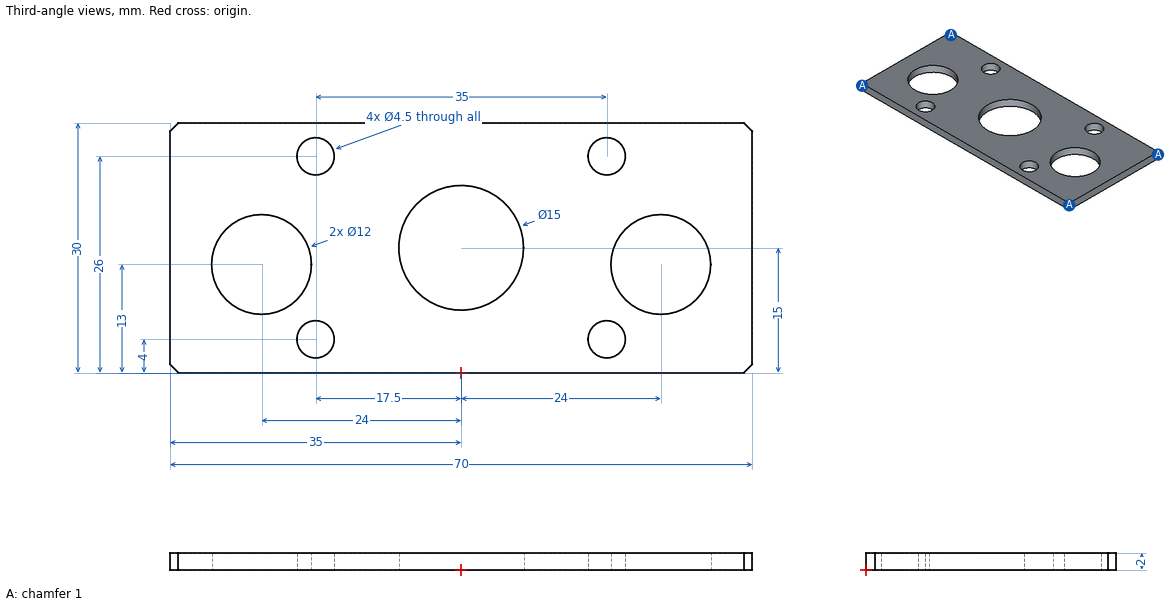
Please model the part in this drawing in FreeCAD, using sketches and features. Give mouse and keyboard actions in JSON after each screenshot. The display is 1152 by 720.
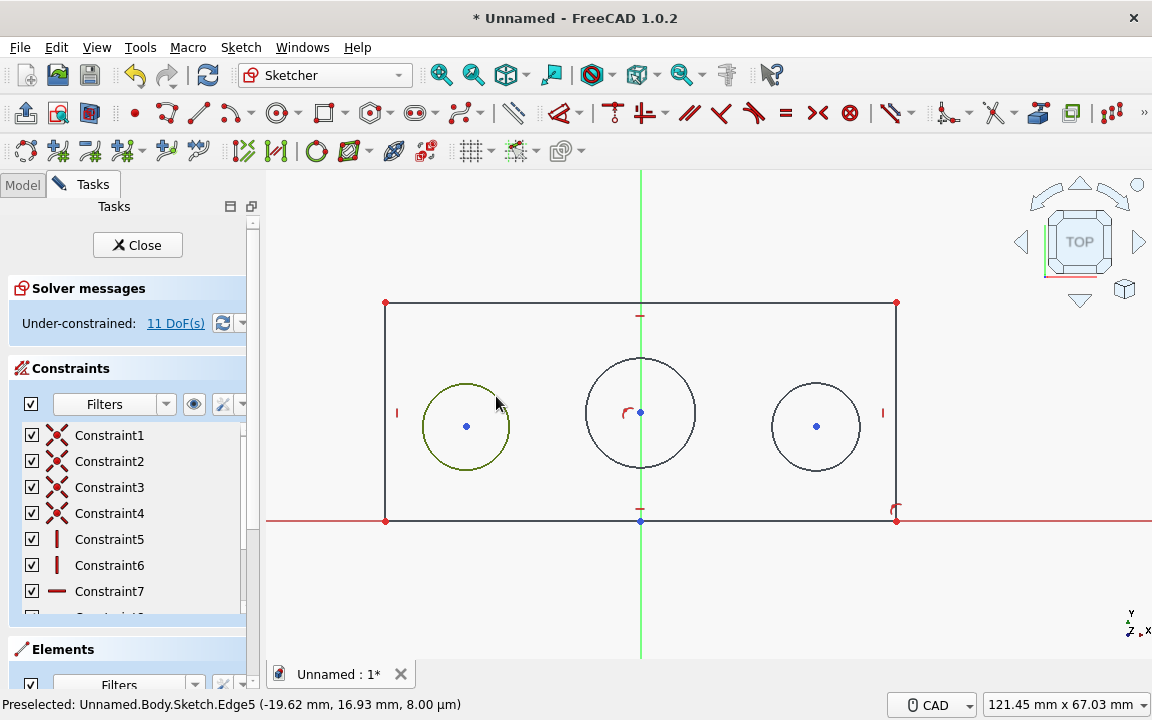
{"action": "left_click", "coordinate": [847, 396]}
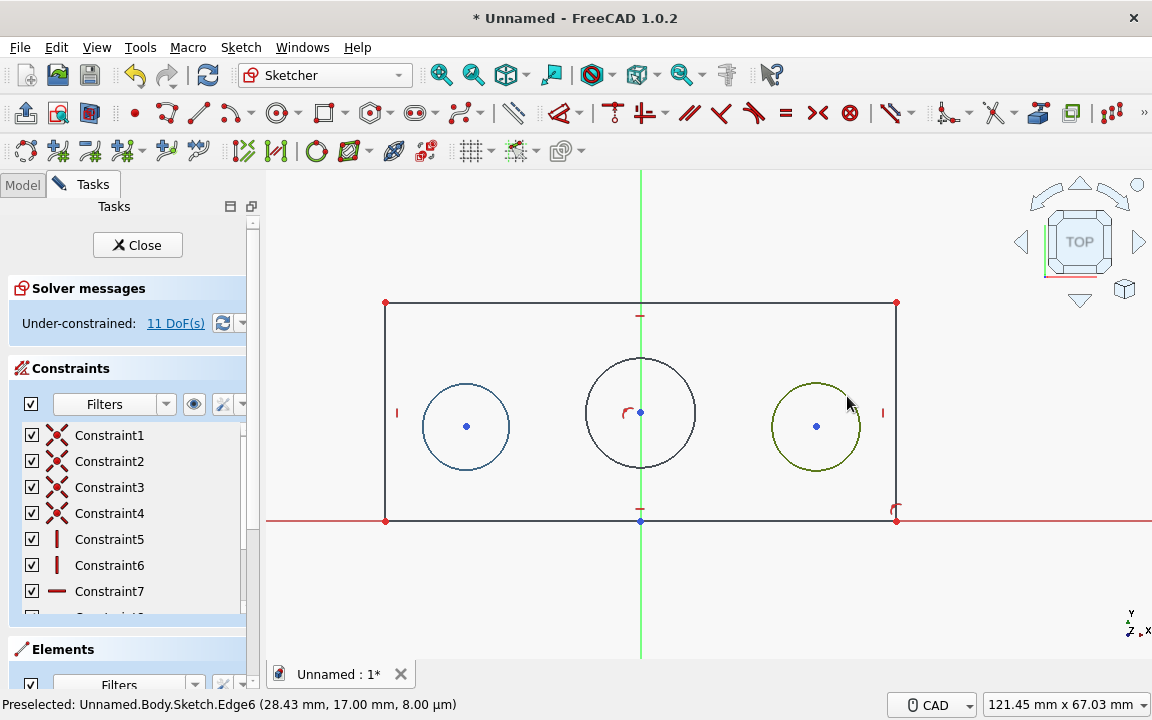
{"action": "left_click", "coordinate": [786, 114]}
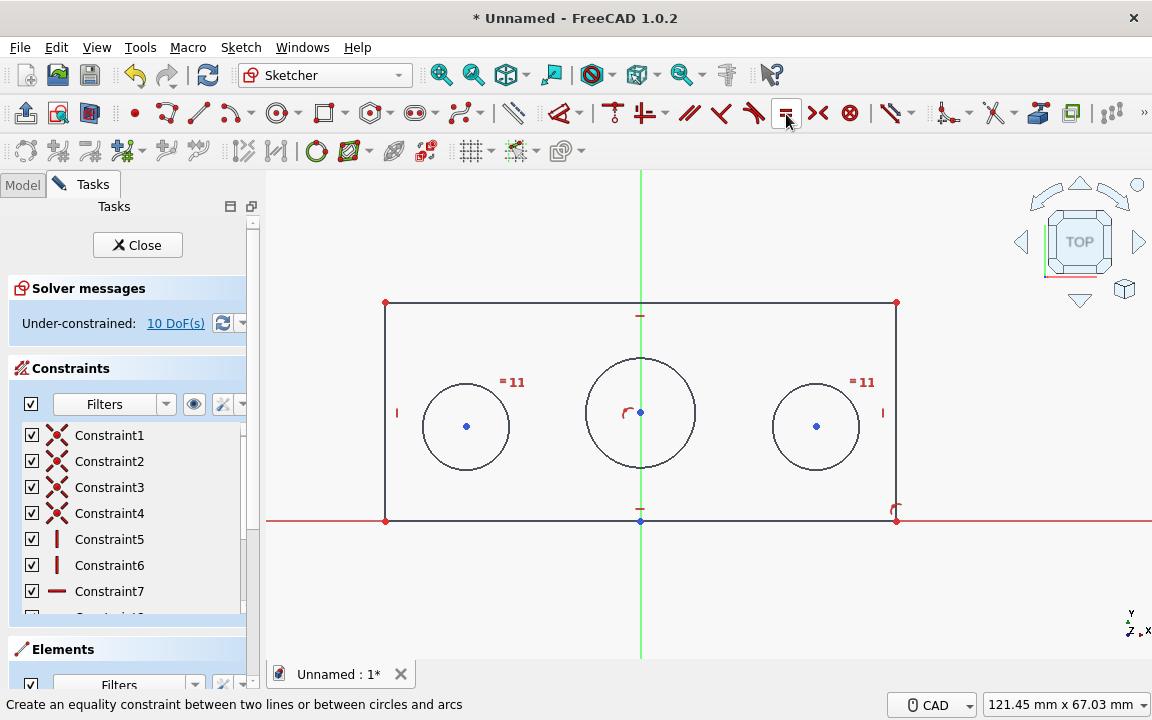
{"action": "left_click", "coordinate": [466, 427]}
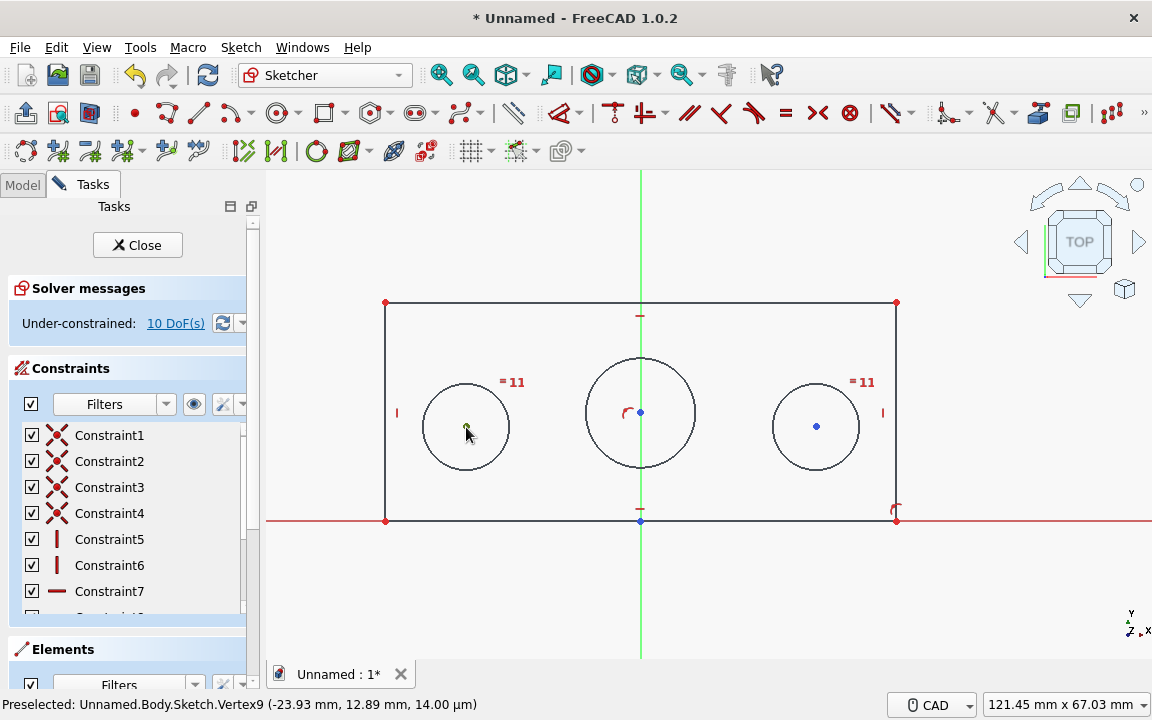
{"action": "left_click", "coordinate": [816, 427]}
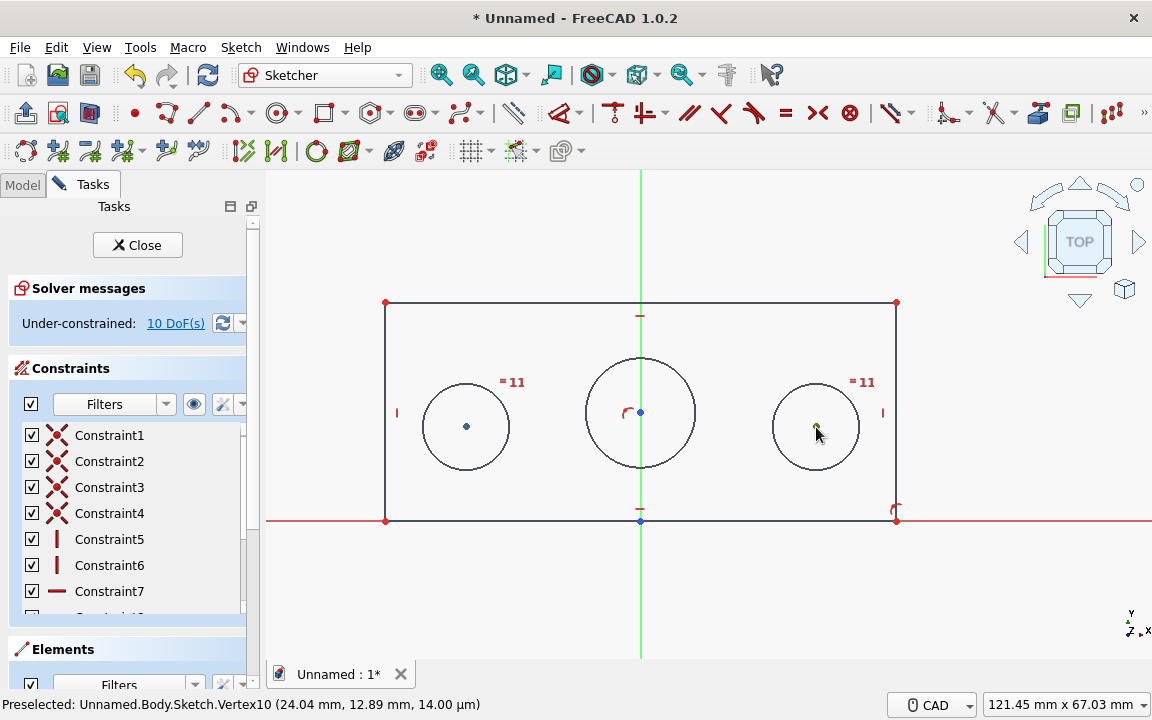
{"action": "key", "text": "h"}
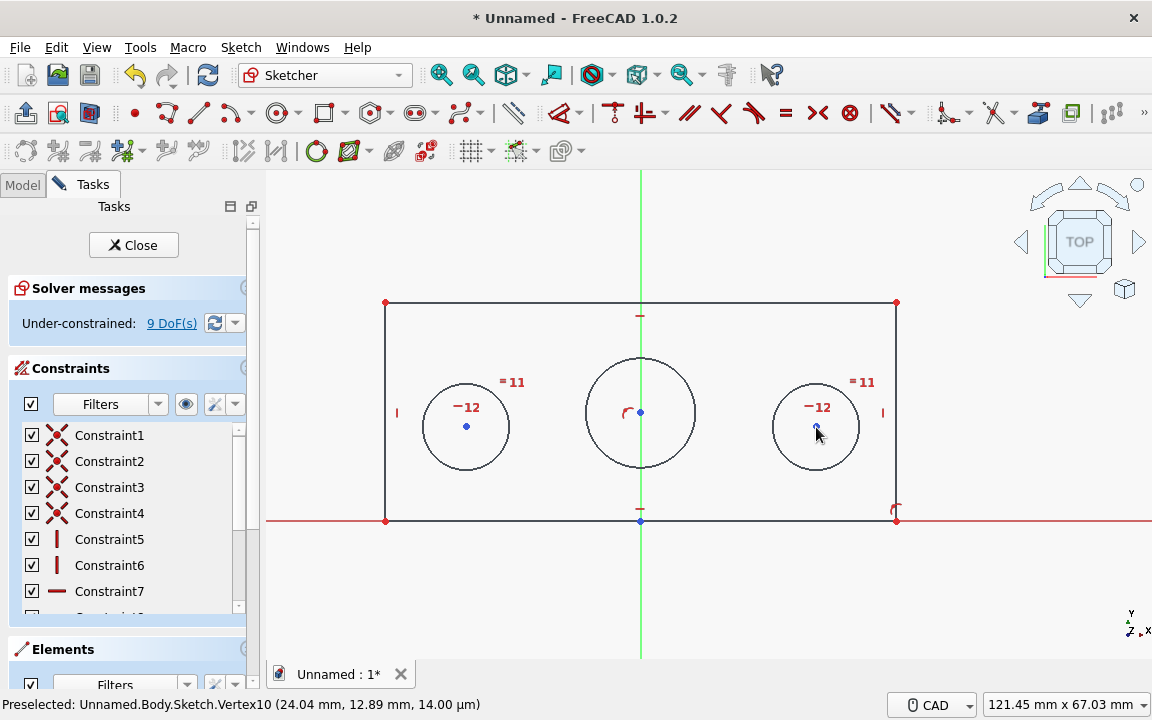
{"action": "left_click", "coordinate": [496, 396]}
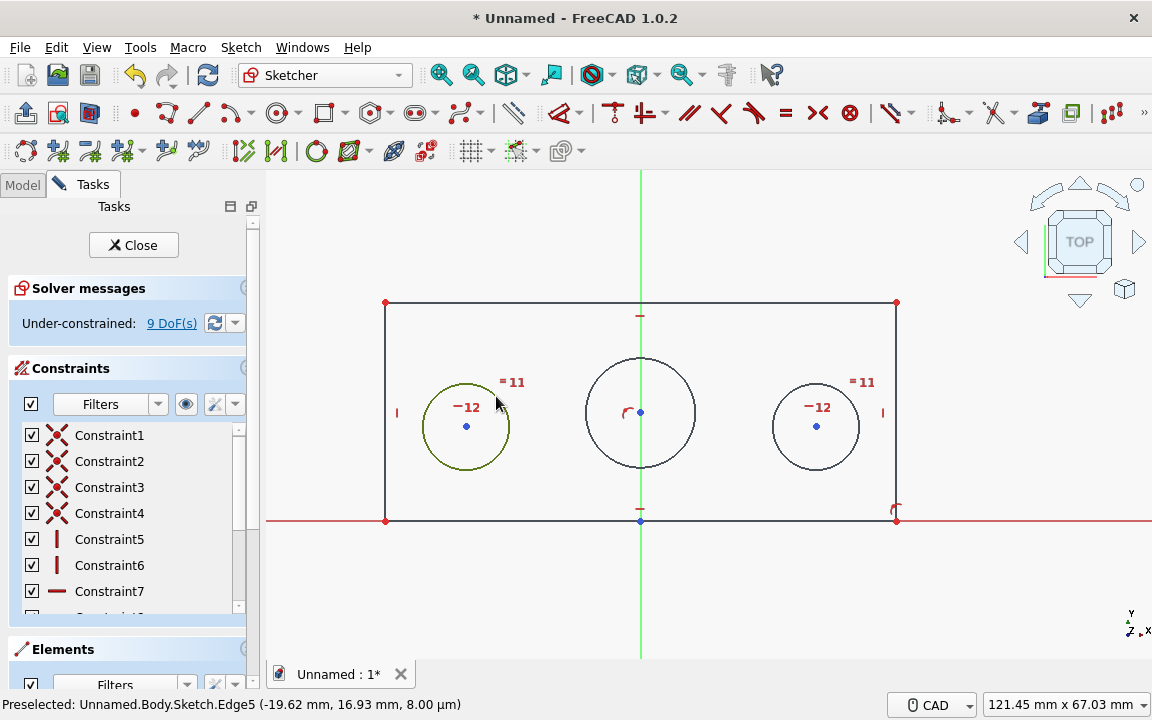
{"action": "left_click", "coordinate": [582, 114]}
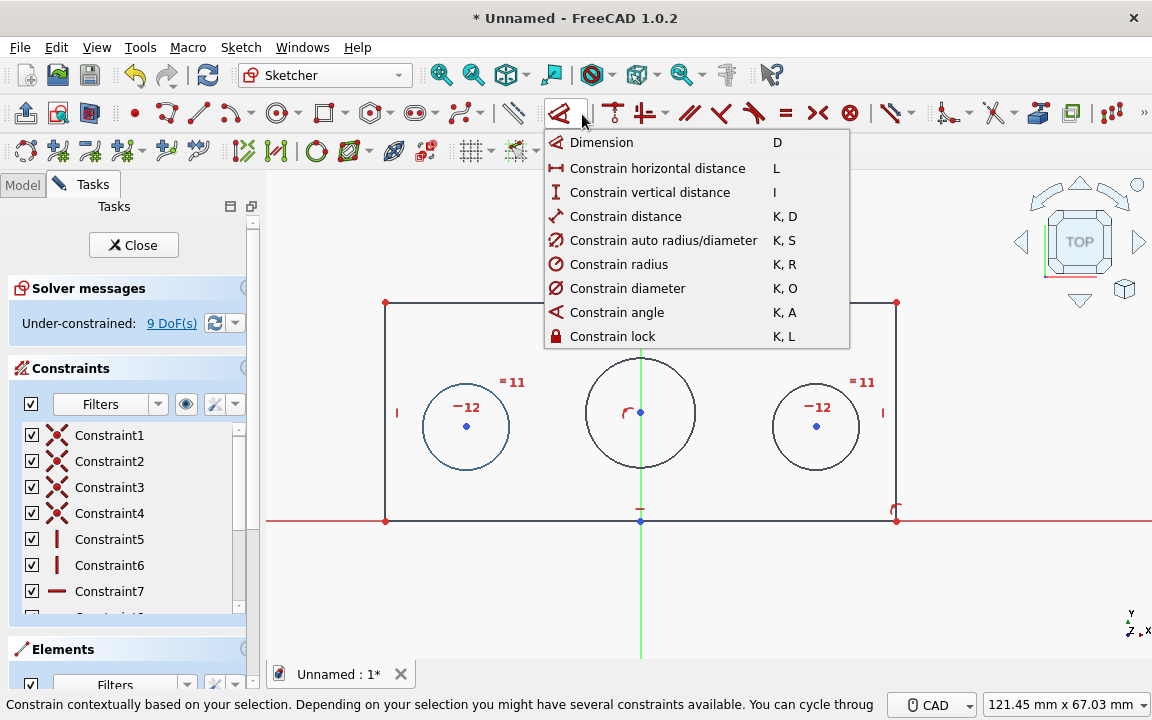
{"action": "left_click", "coordinate": [697, 288]}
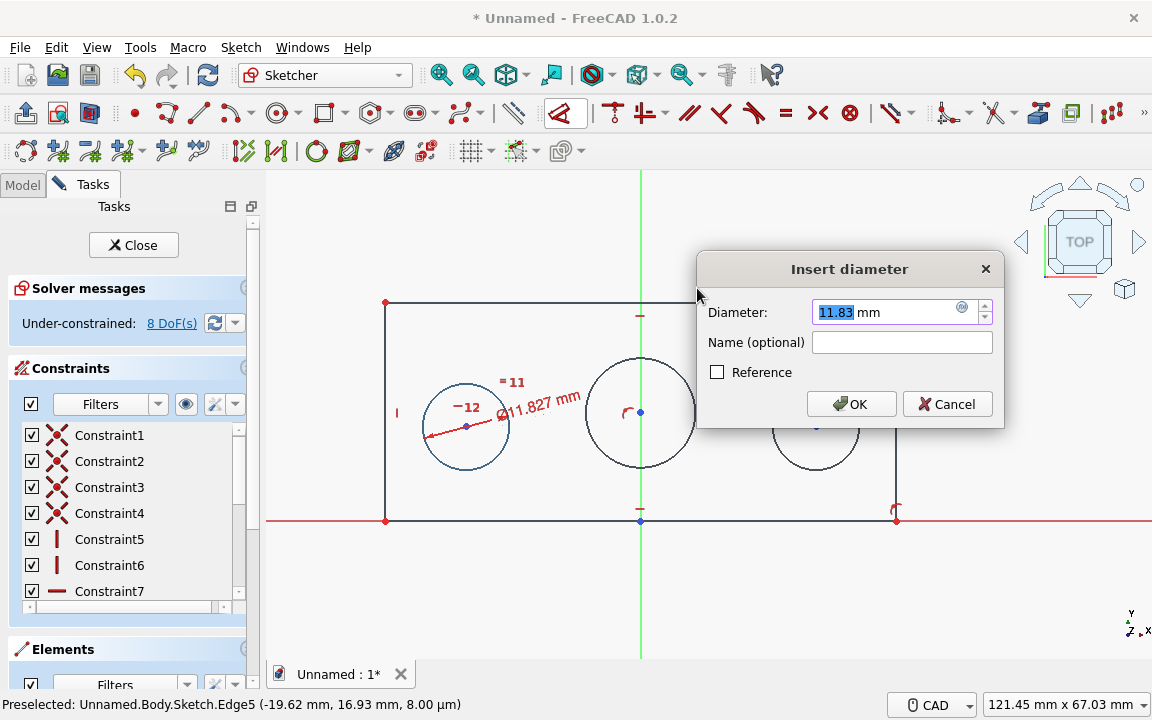
{"action": "type", "text": "12"}
{"action": "key", "text": "Return"}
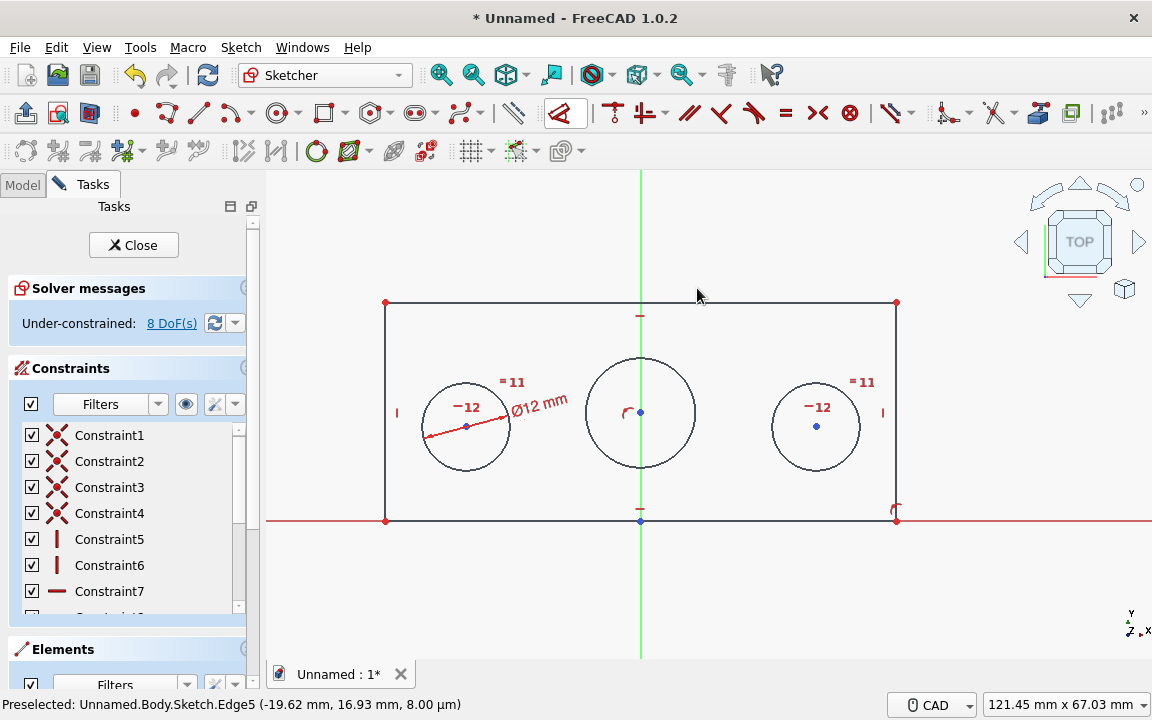
{"action": "left_click", "coordinate": [679, 374]}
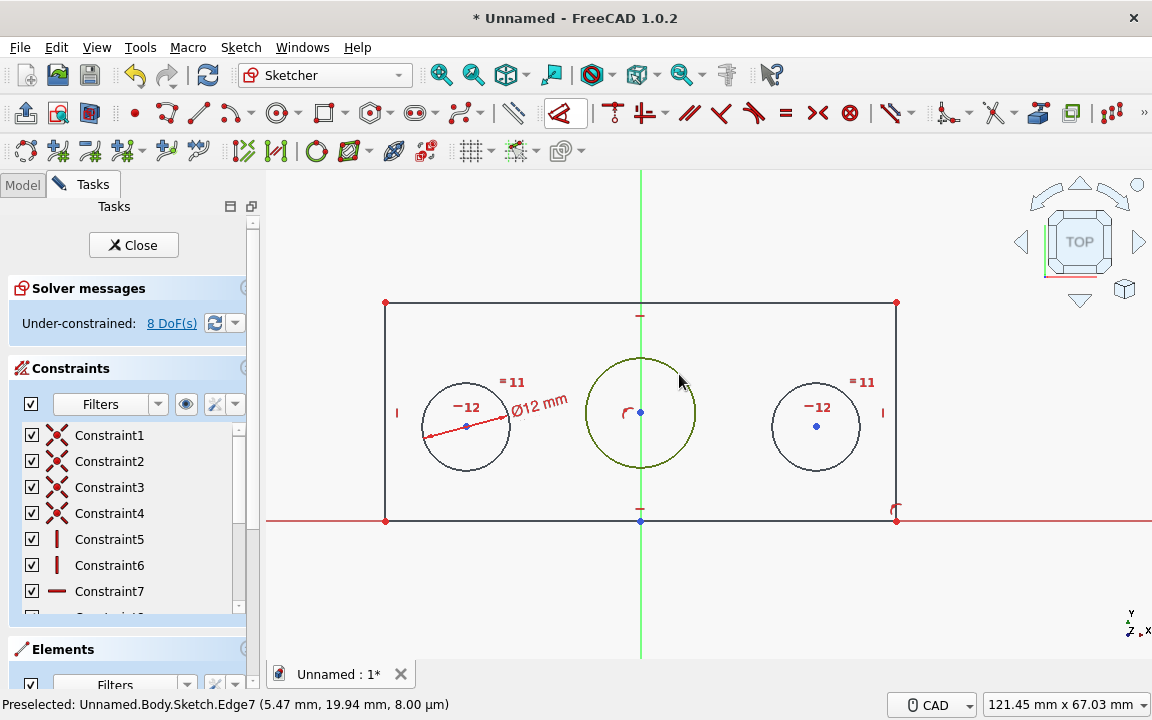
{"action": "left_click", "coordinate": [582, 114]}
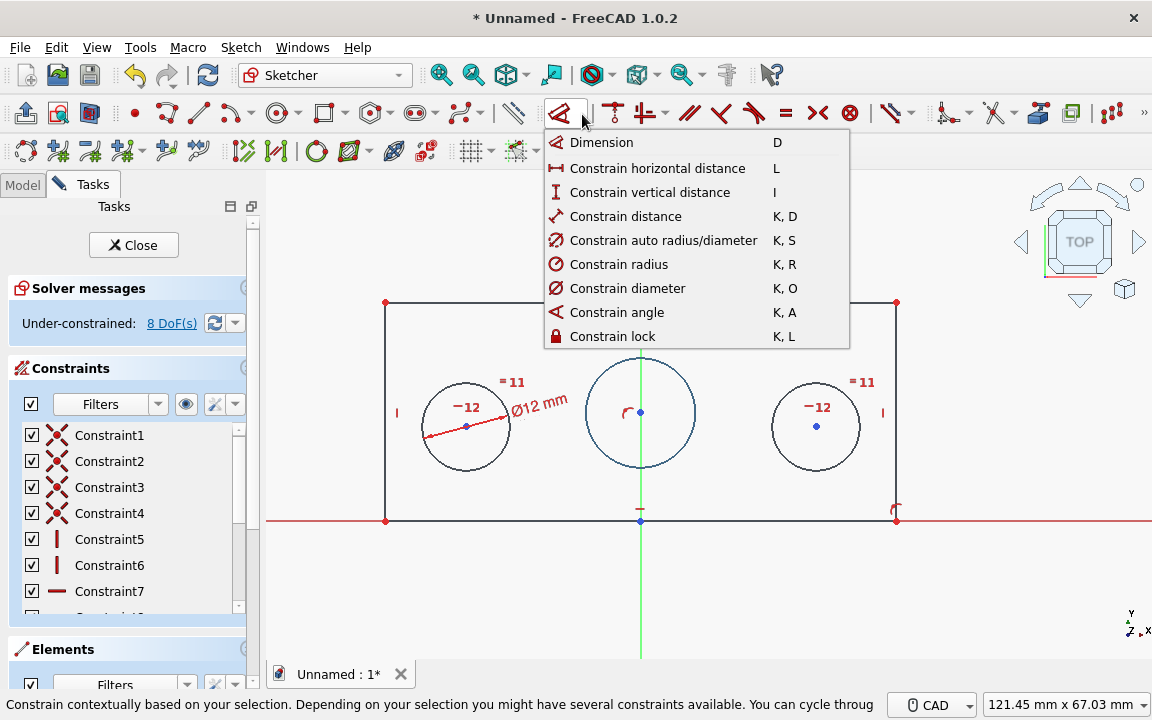
{"action": "left_click", "coordinate": [697, 288]}